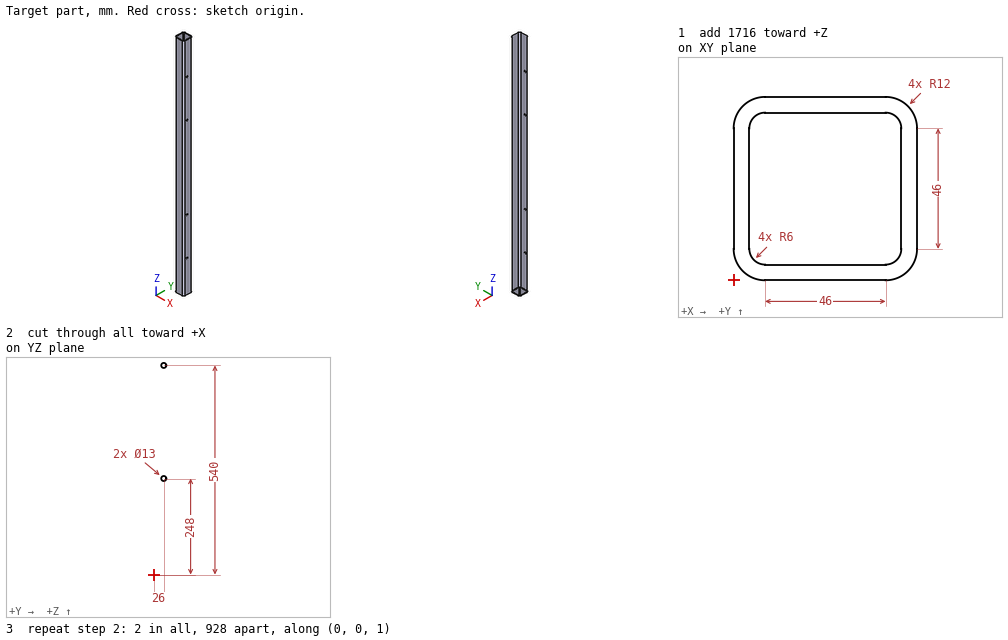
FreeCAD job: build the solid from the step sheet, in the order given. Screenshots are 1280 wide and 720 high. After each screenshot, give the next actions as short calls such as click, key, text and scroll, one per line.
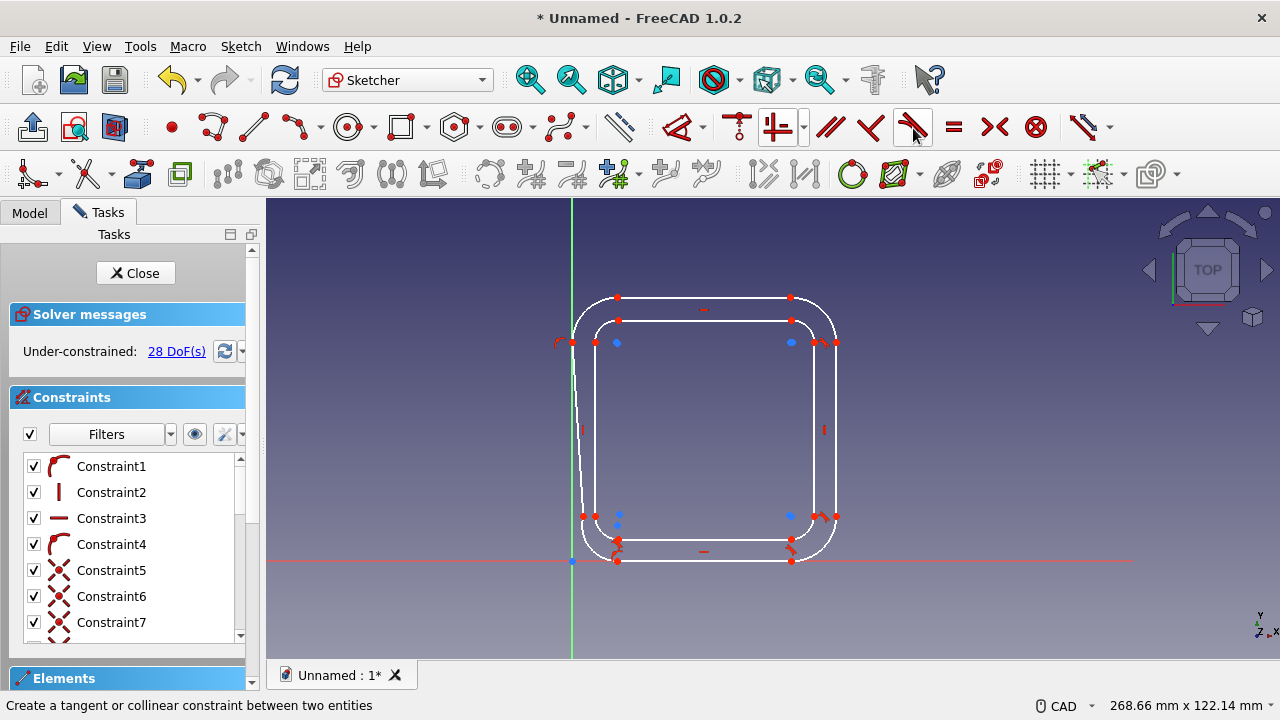
click(739, 298)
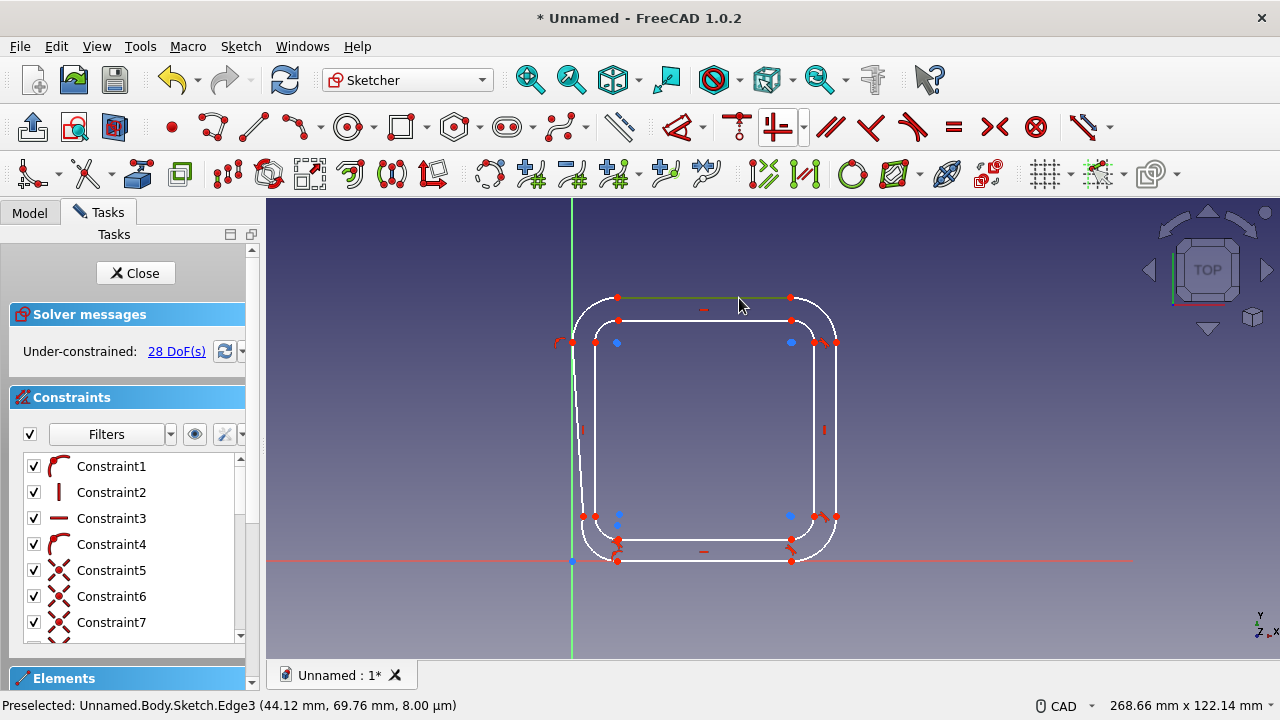
click(831, 322)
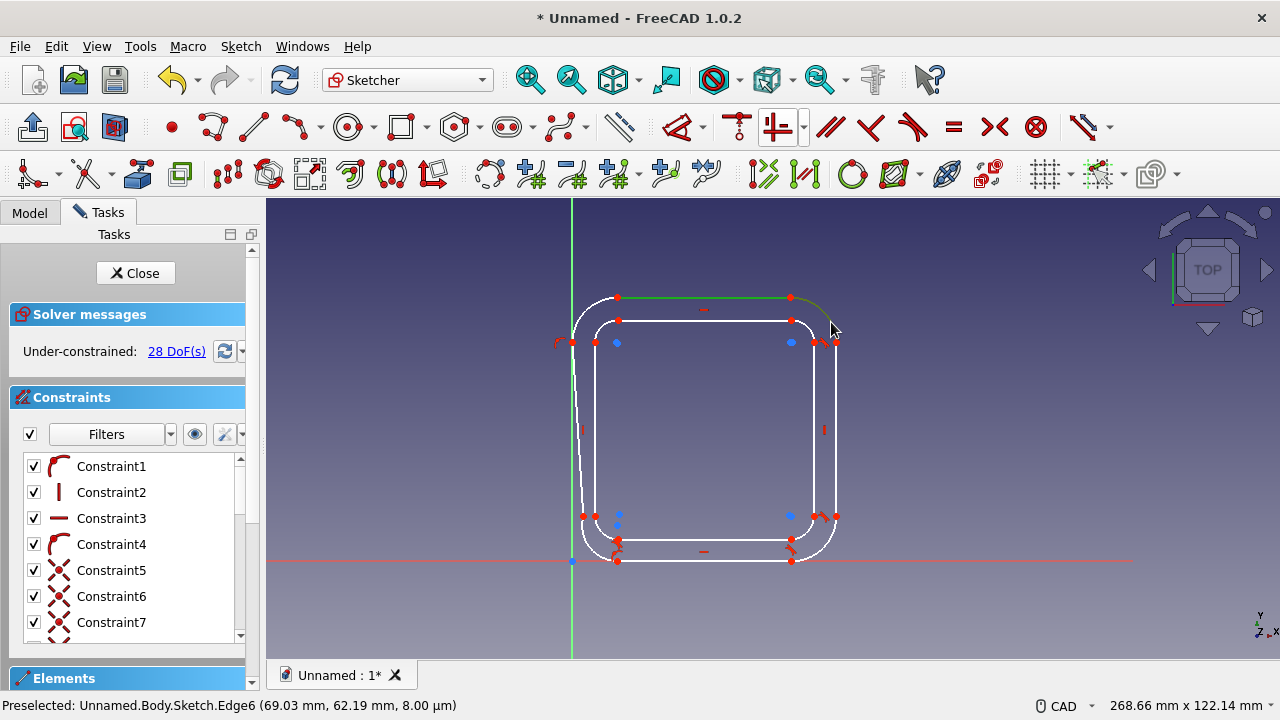
click(913, 128)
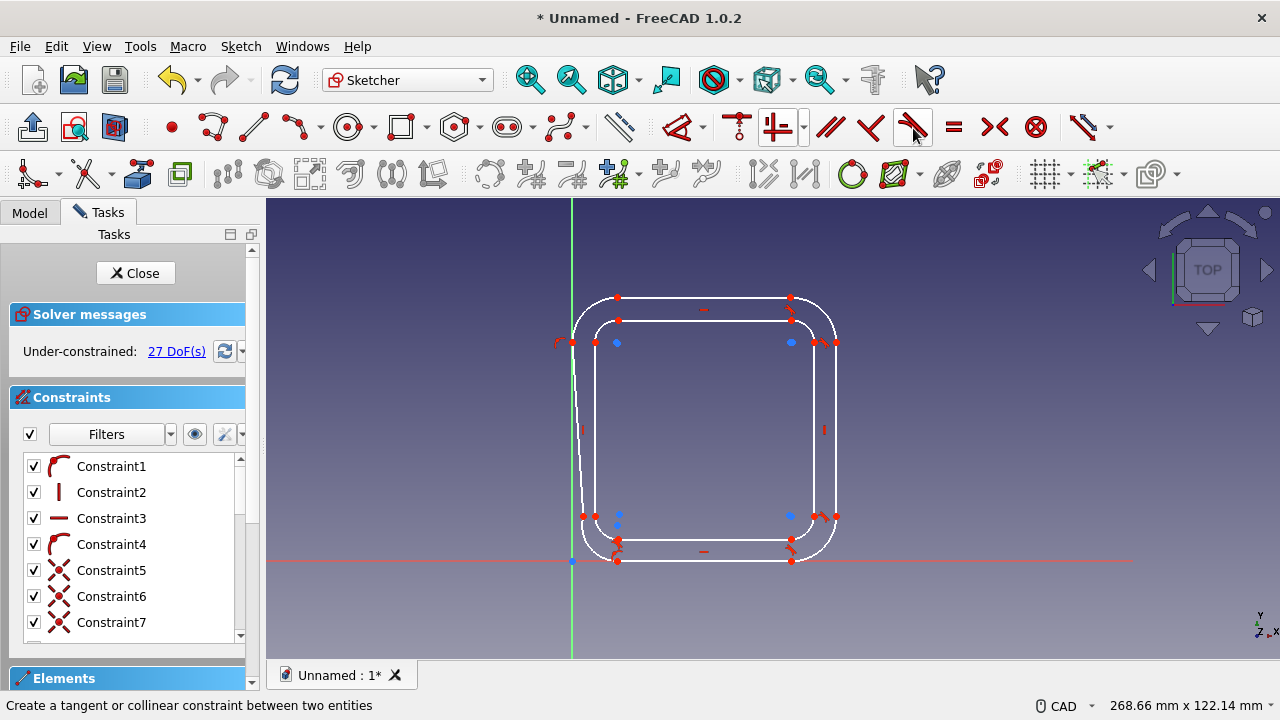
click(739, 298)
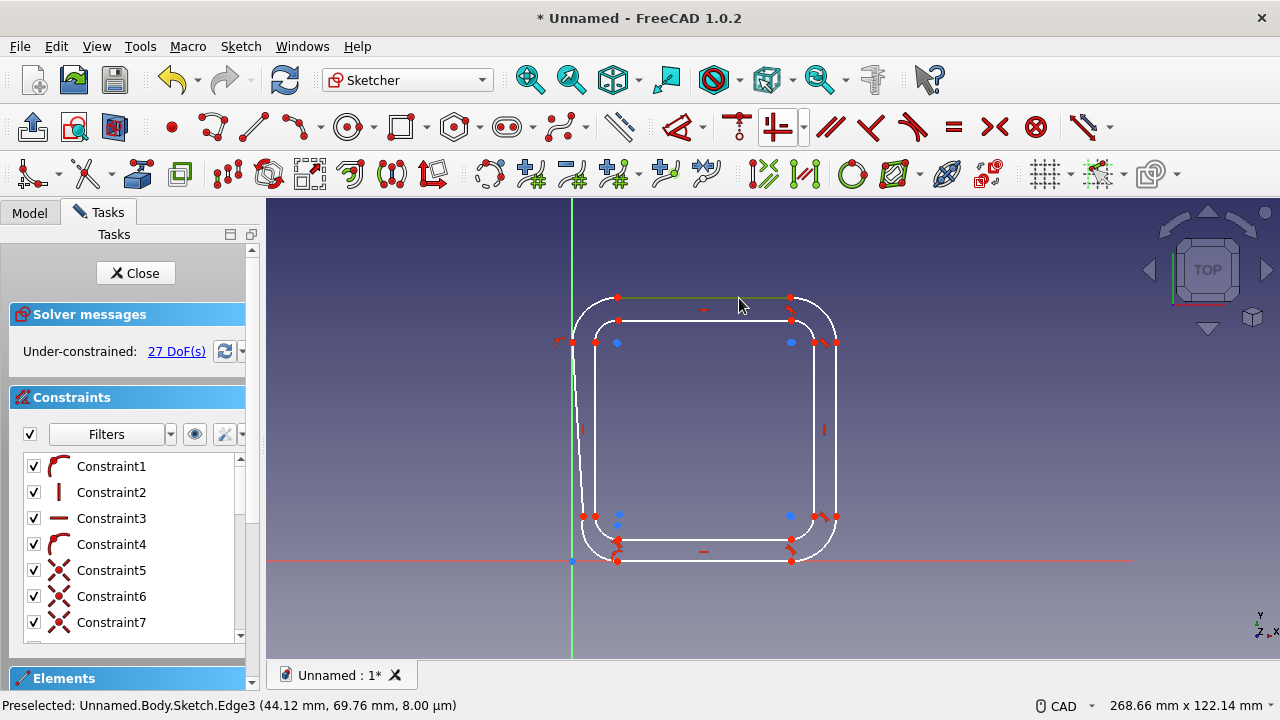
click(597, 303)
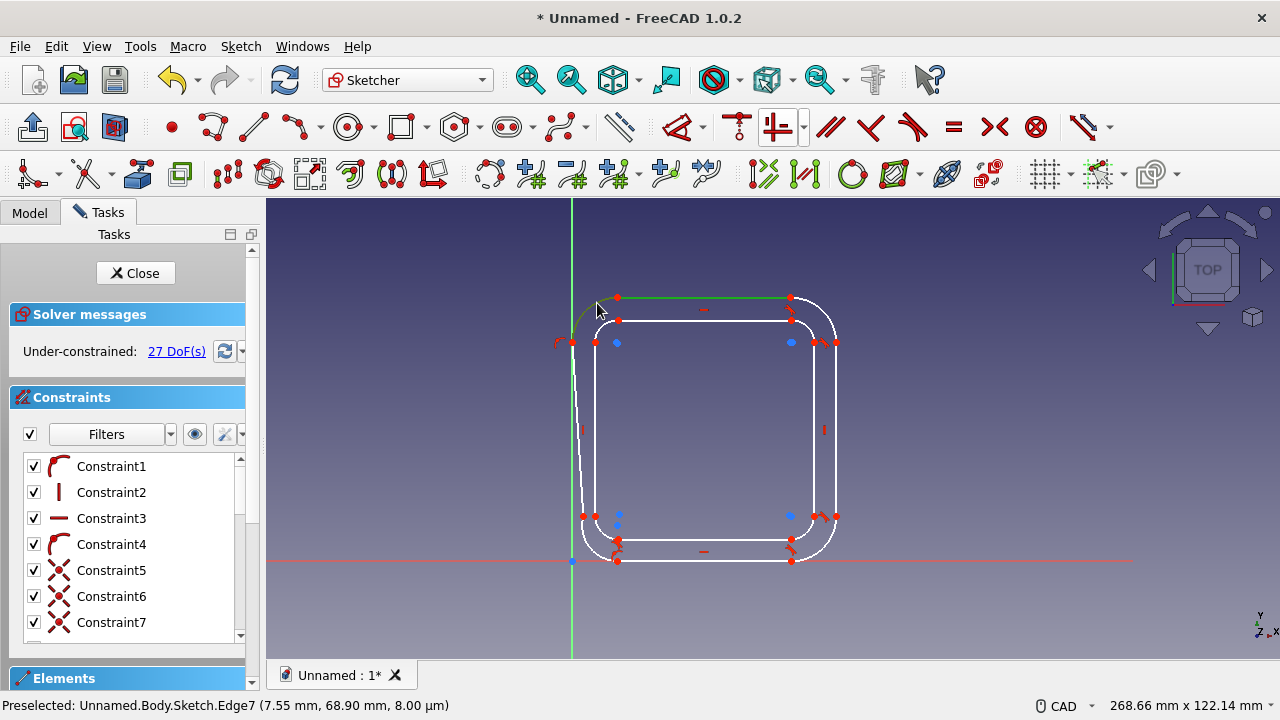
click(913, 128)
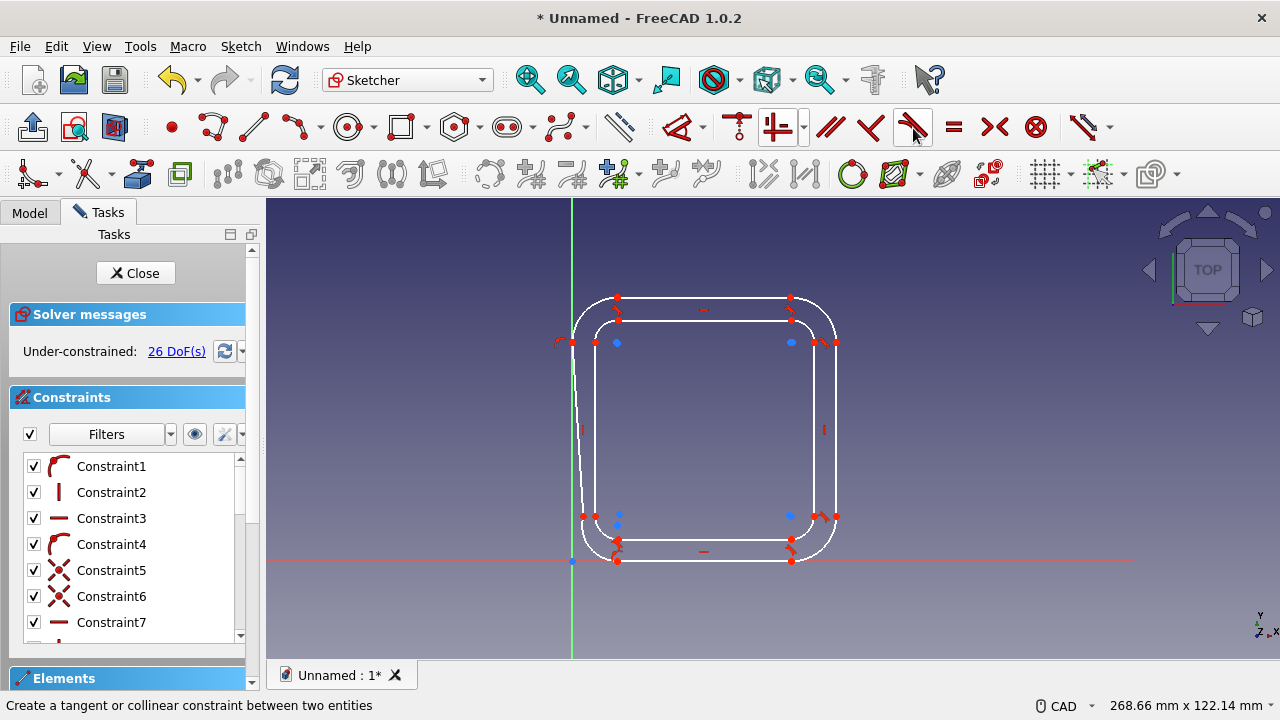
click(576, 395)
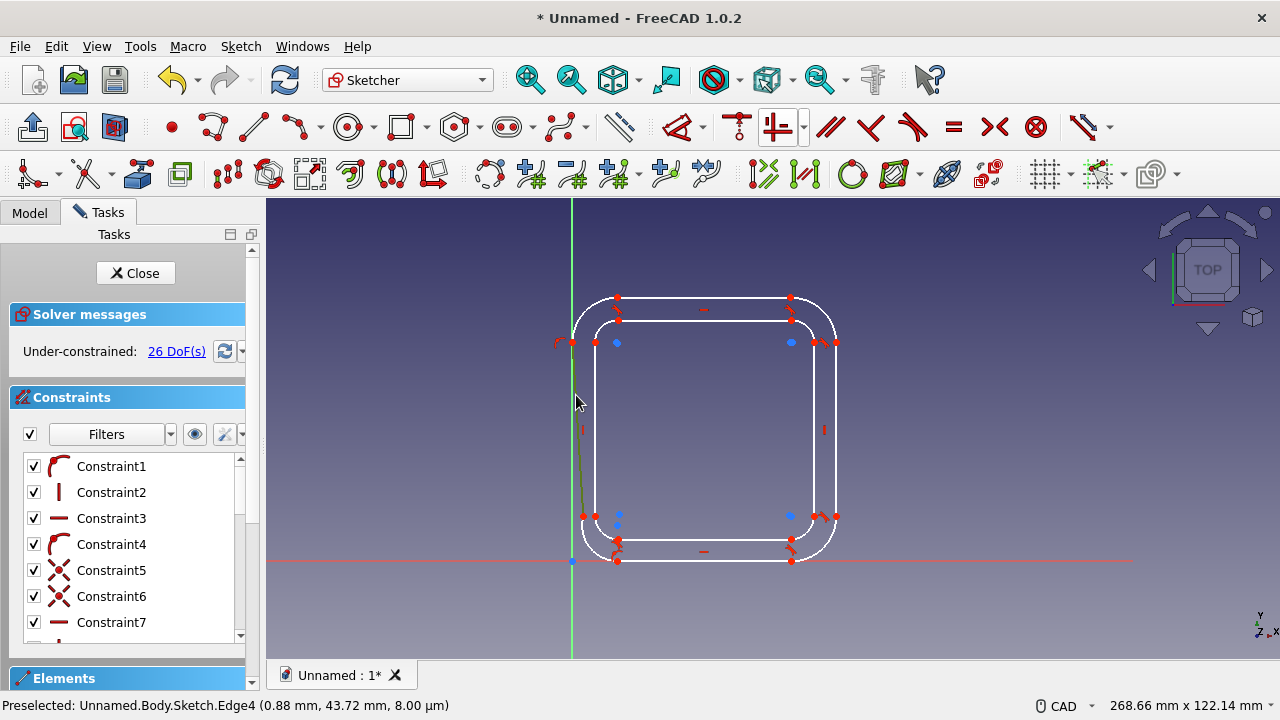
click(597, 303)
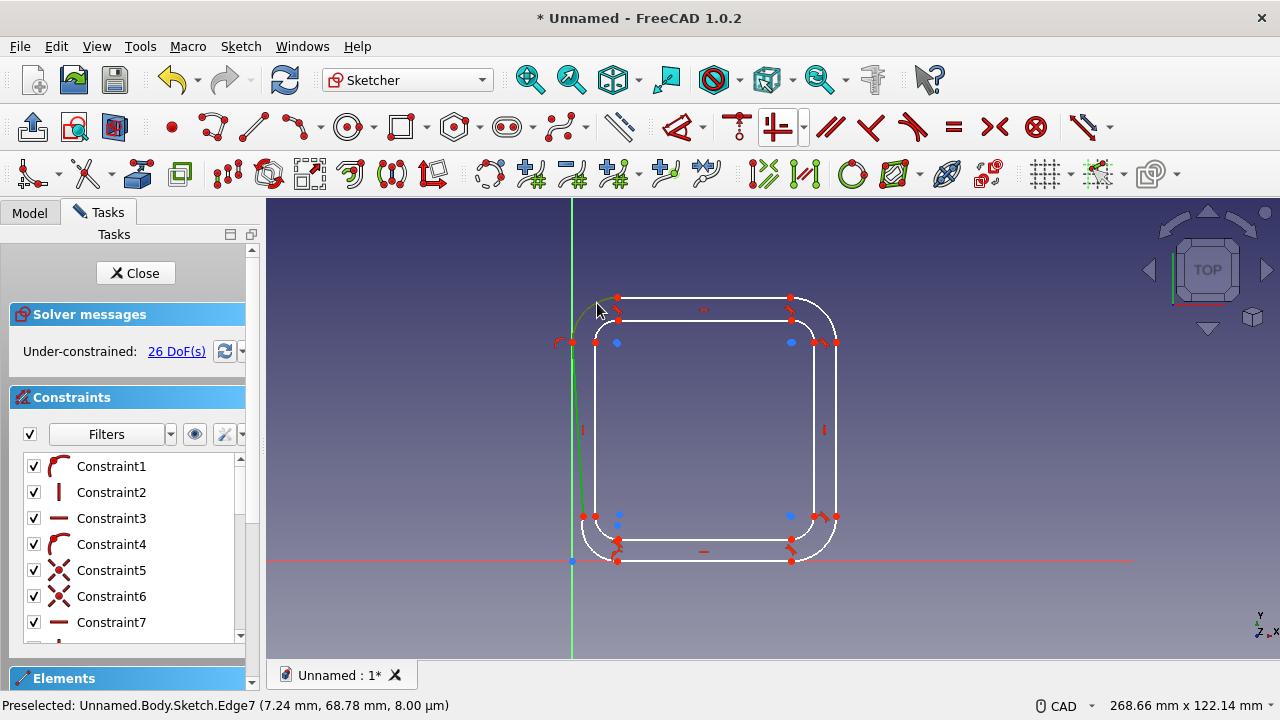
click(913, 128)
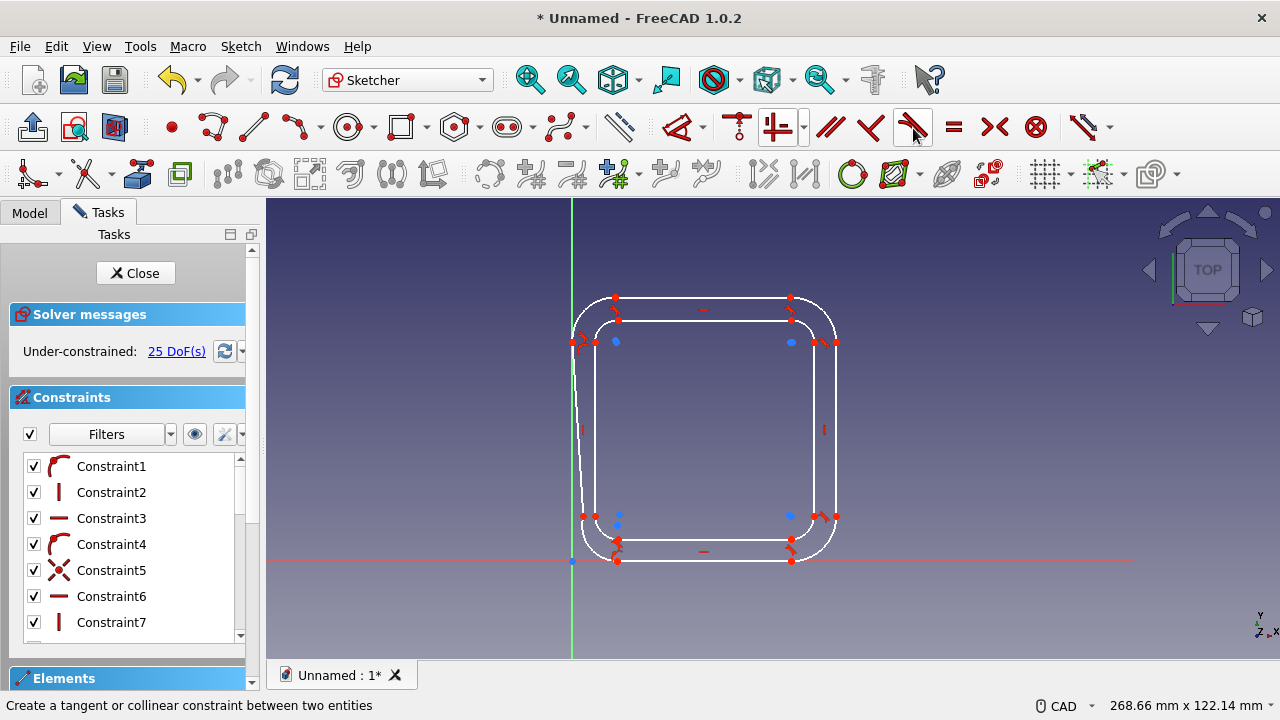
click(576, 395)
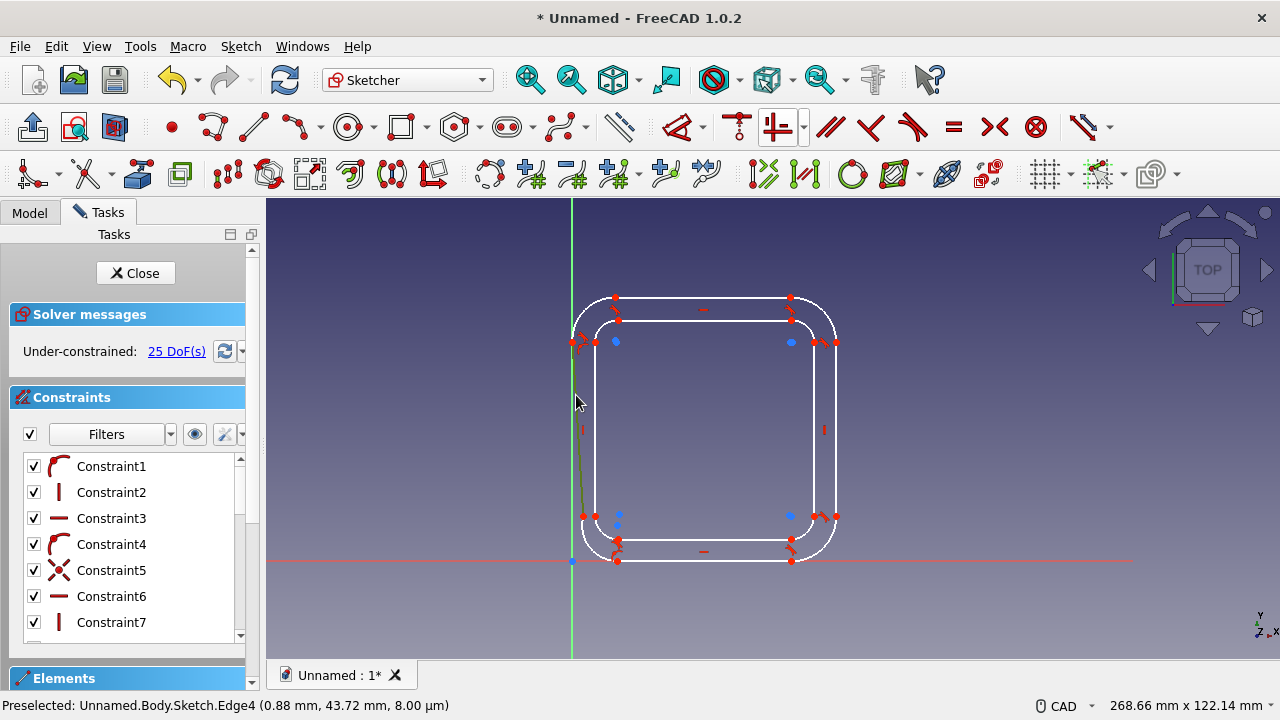
scroll(584, 536, up, 2)